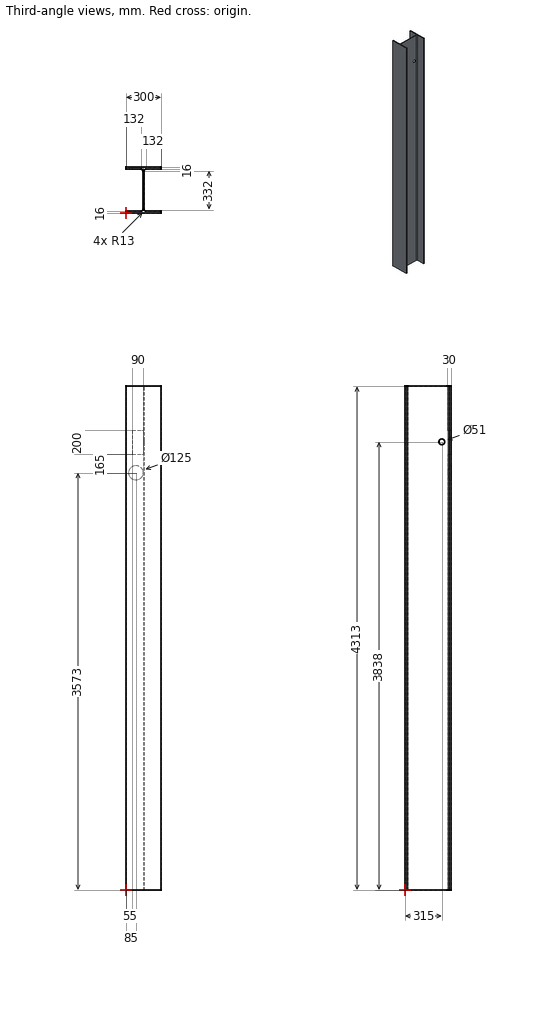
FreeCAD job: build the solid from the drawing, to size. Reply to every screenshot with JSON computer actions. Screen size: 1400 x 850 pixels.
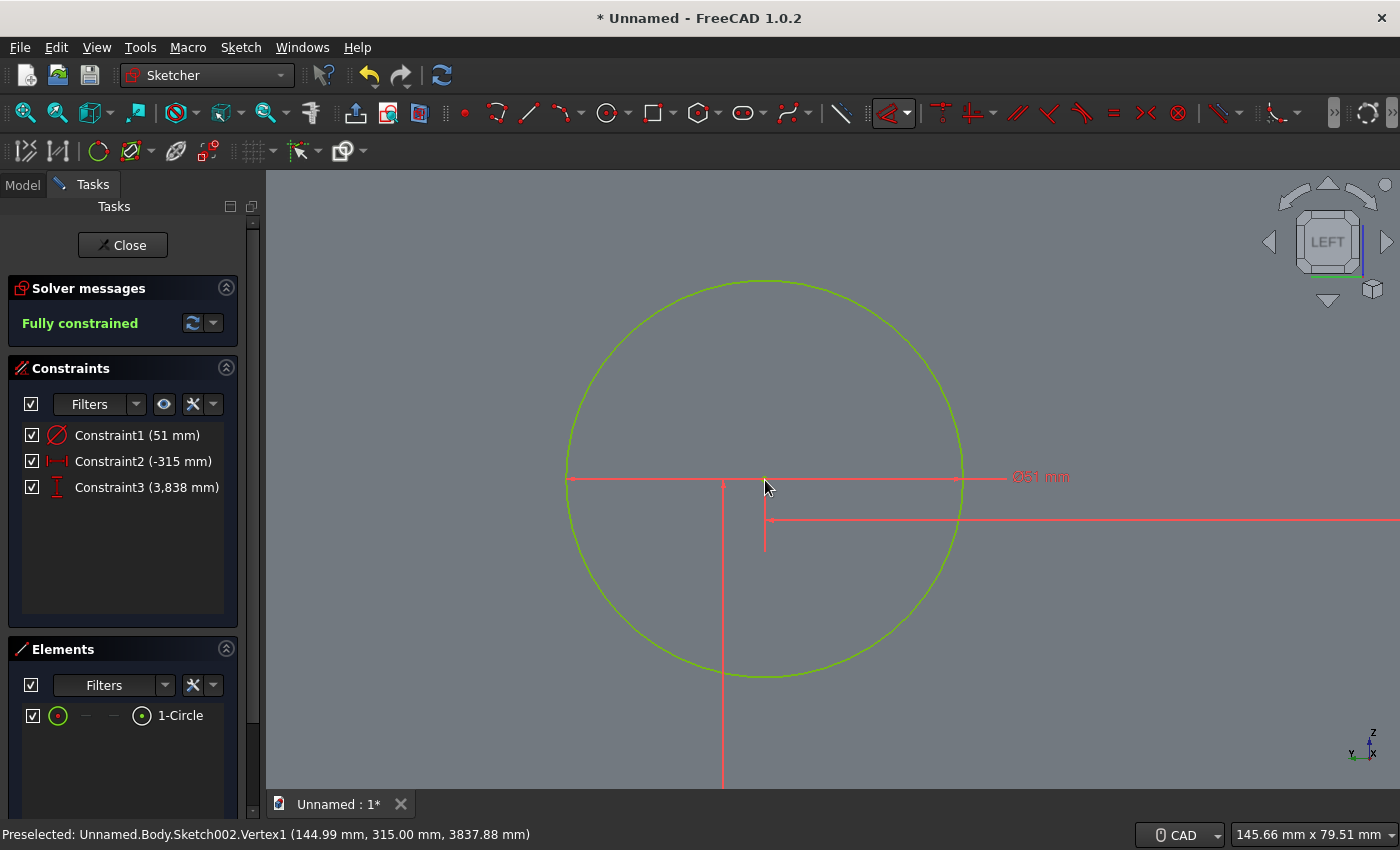
{"action": "left_click", "coordinate": [123, 245]}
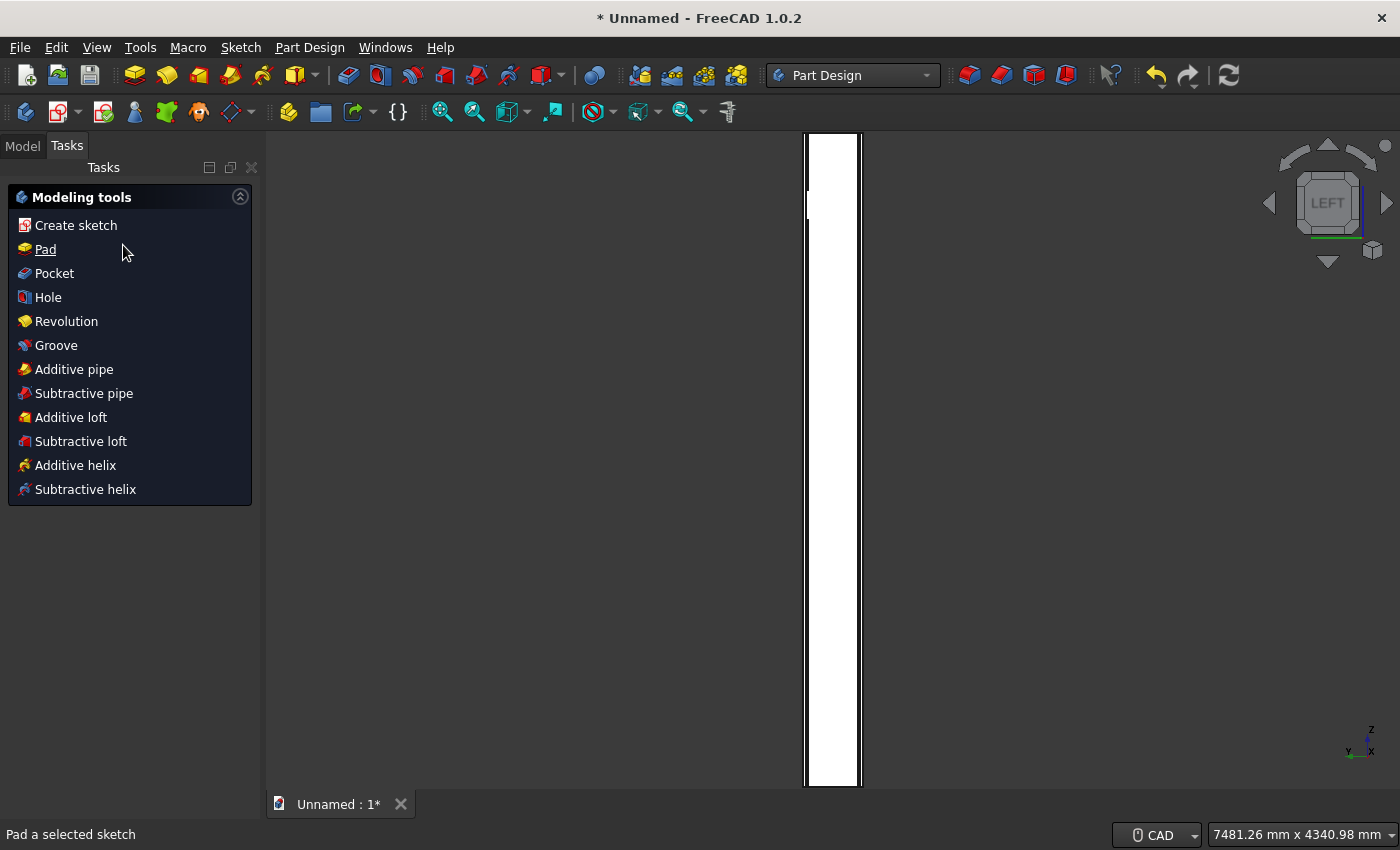
{"action": "left_click", "coordinate": [350, 76]}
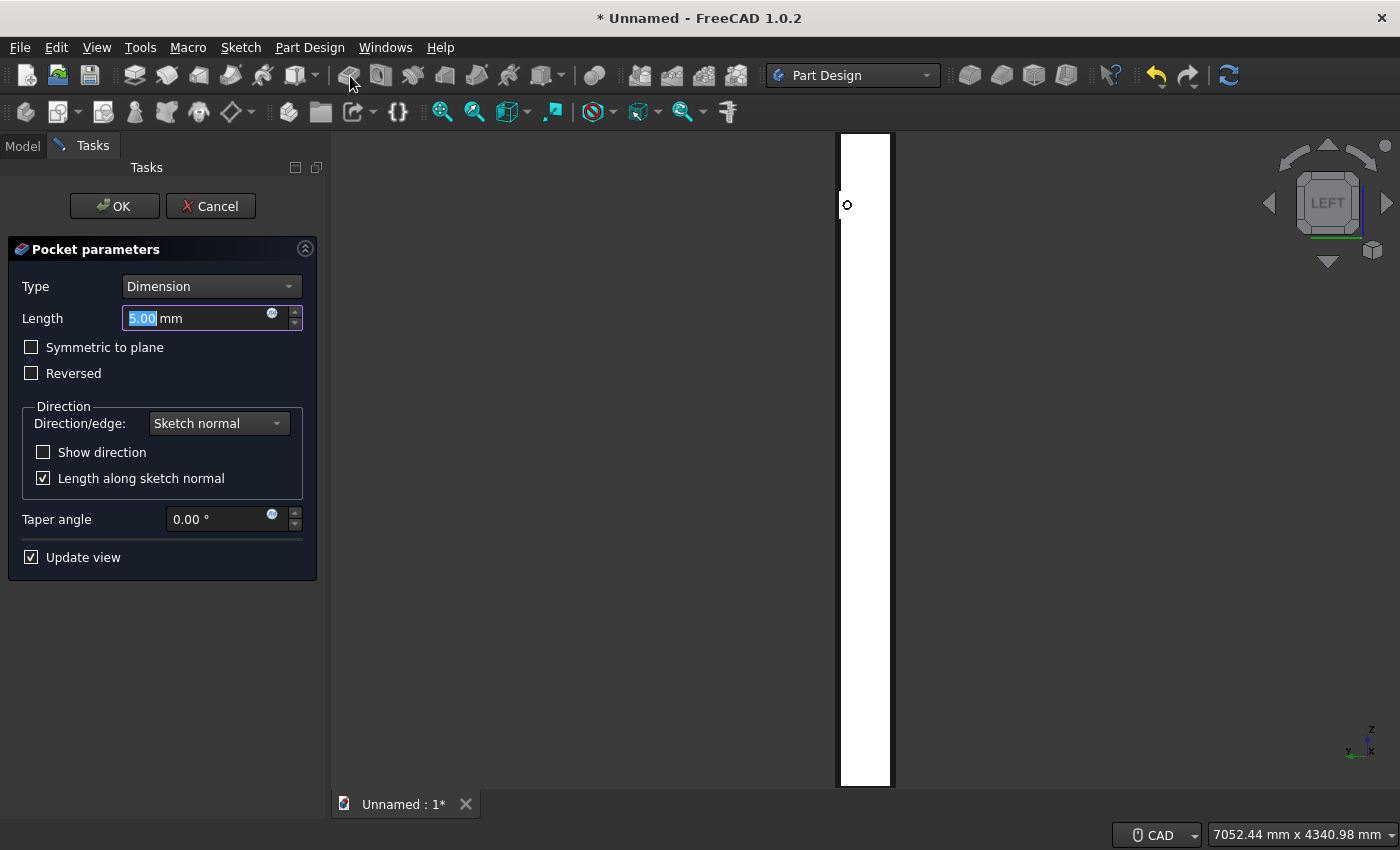
{"action": "left_click", "coordinate": [212, 286]}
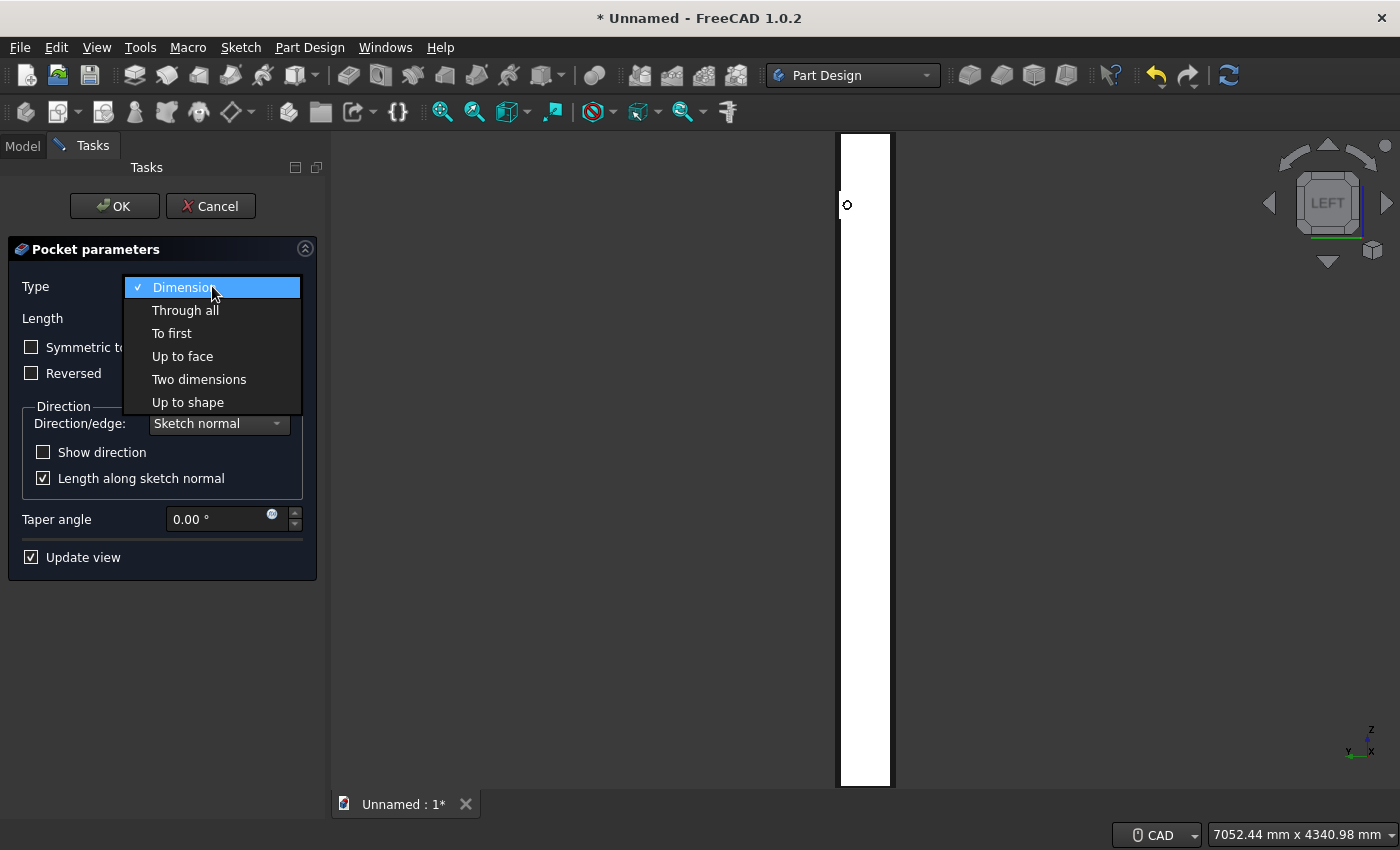
{"action": "left_click", "coordinate": [212, 334]}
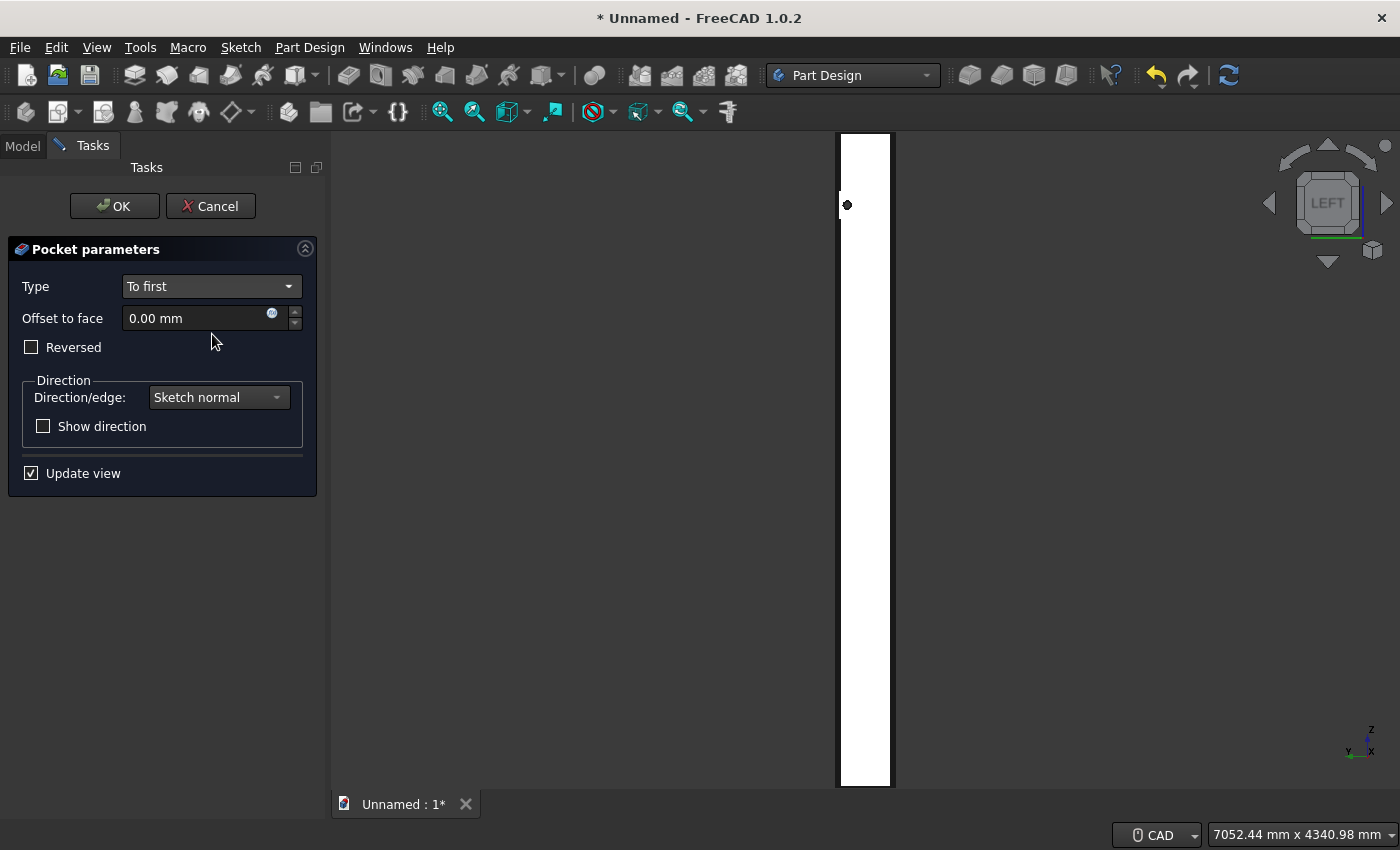
{"action": "left_click", "coordinate": [115, 206]}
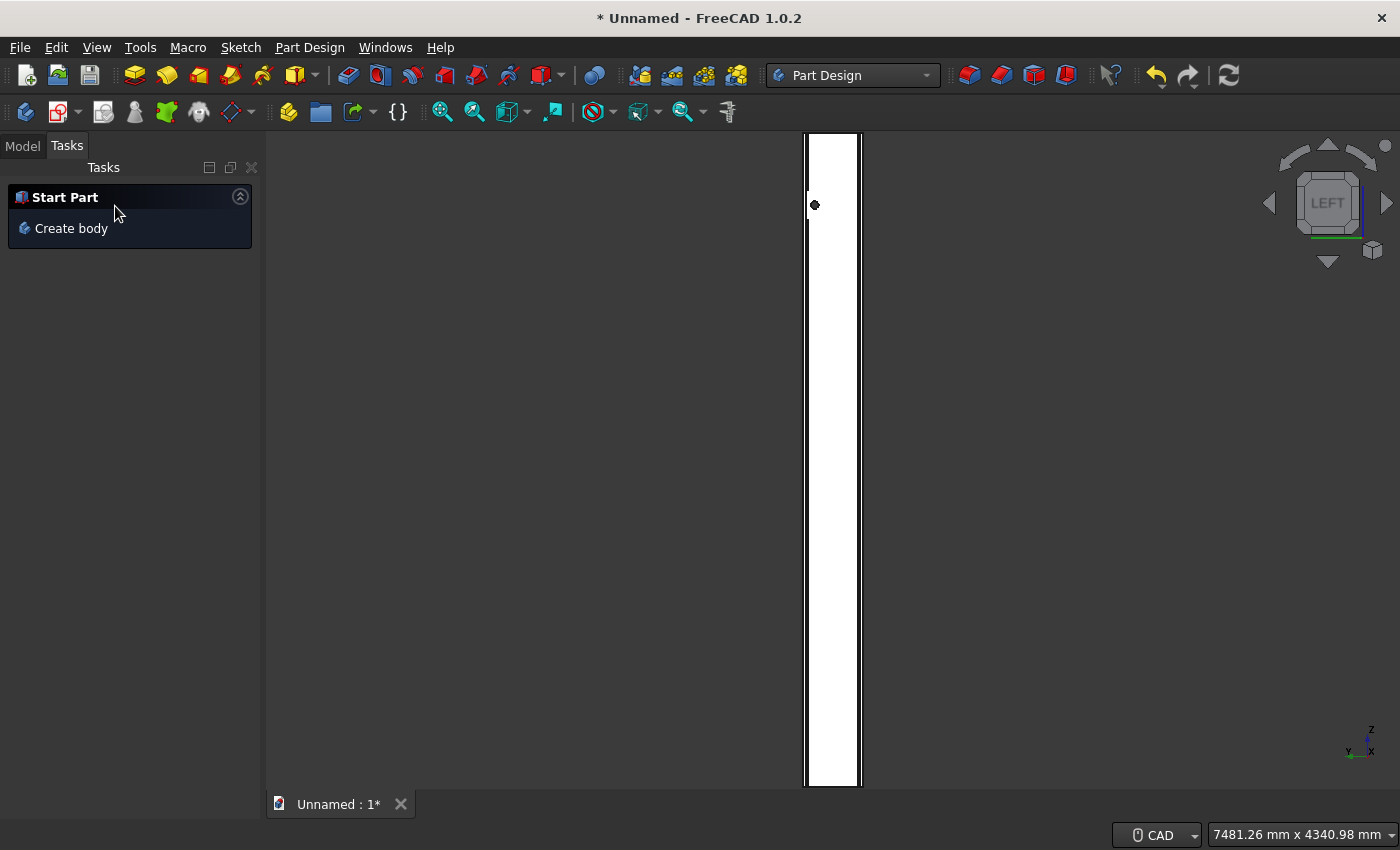
{"action": "key", "text": "0"}